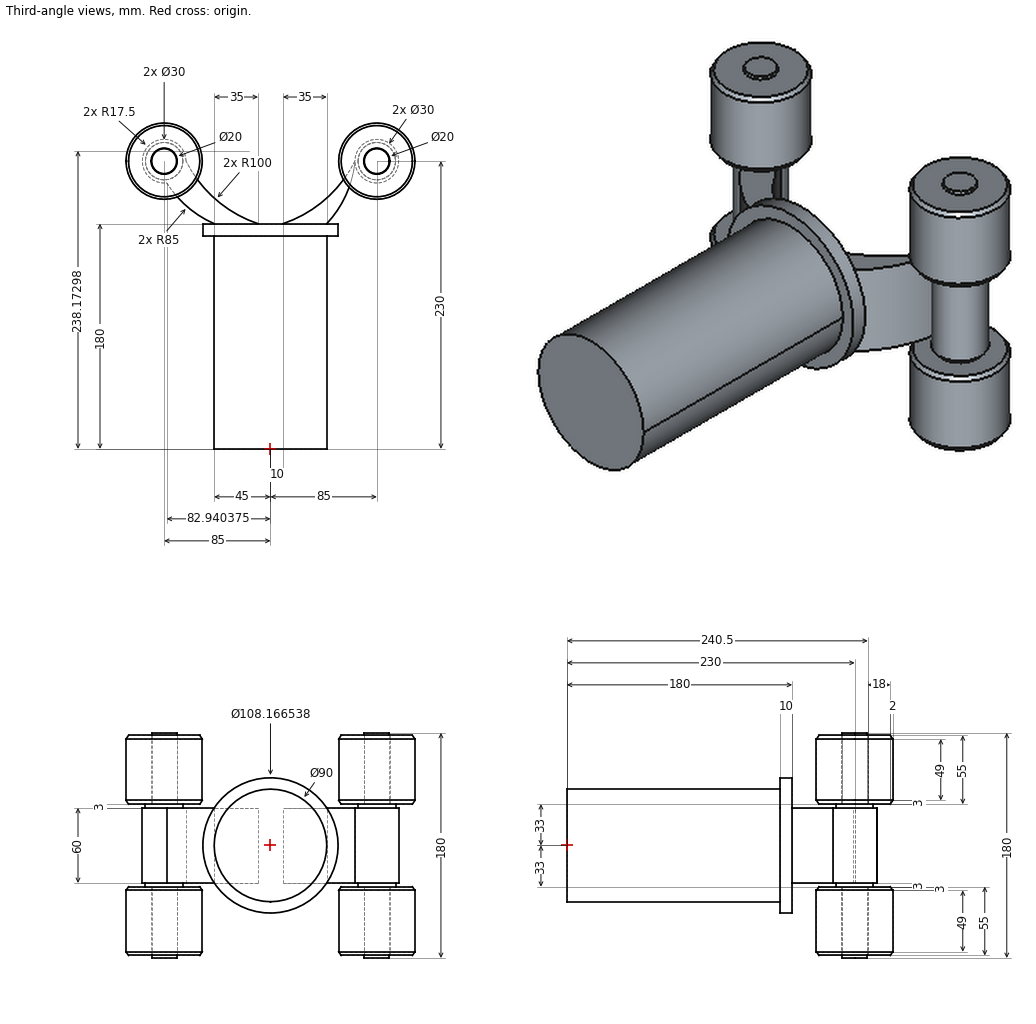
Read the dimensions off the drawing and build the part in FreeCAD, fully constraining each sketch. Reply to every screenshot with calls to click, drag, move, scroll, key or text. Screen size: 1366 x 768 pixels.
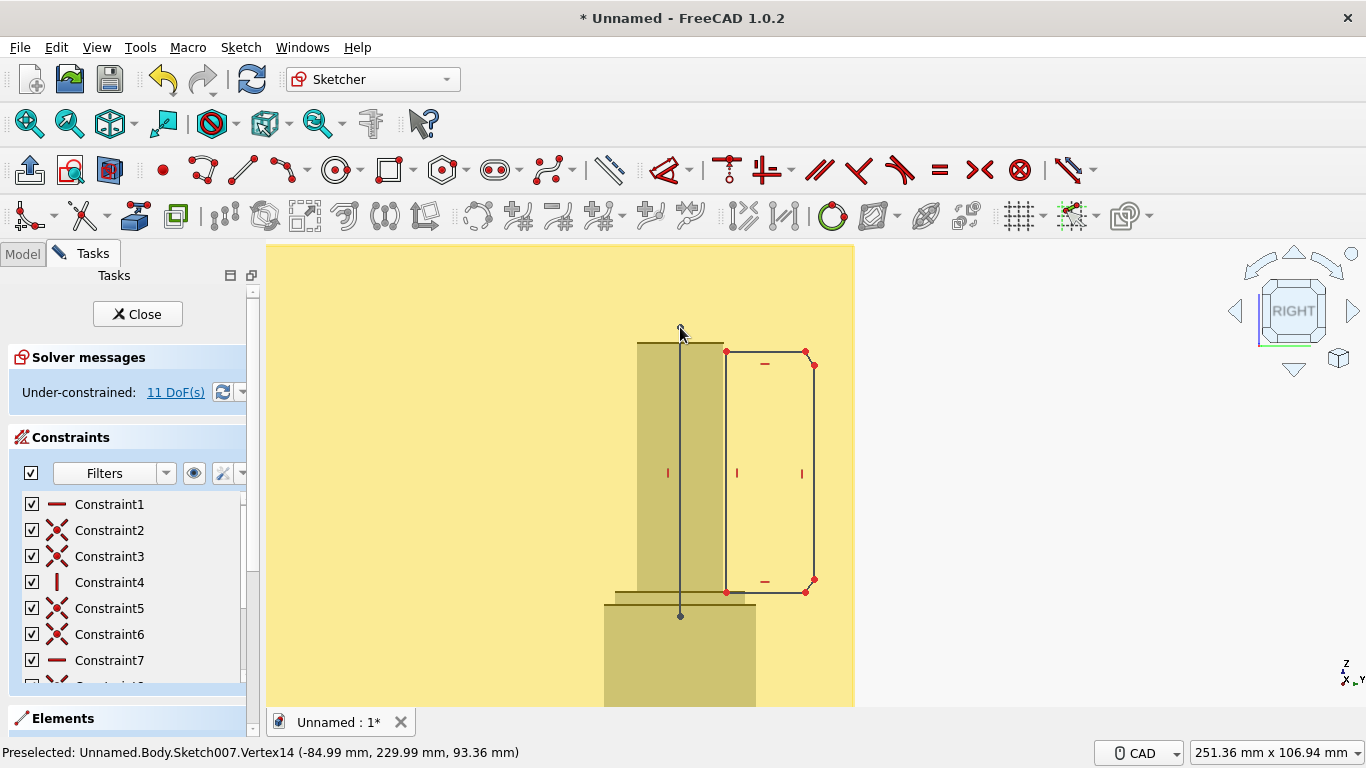
click(680, 530)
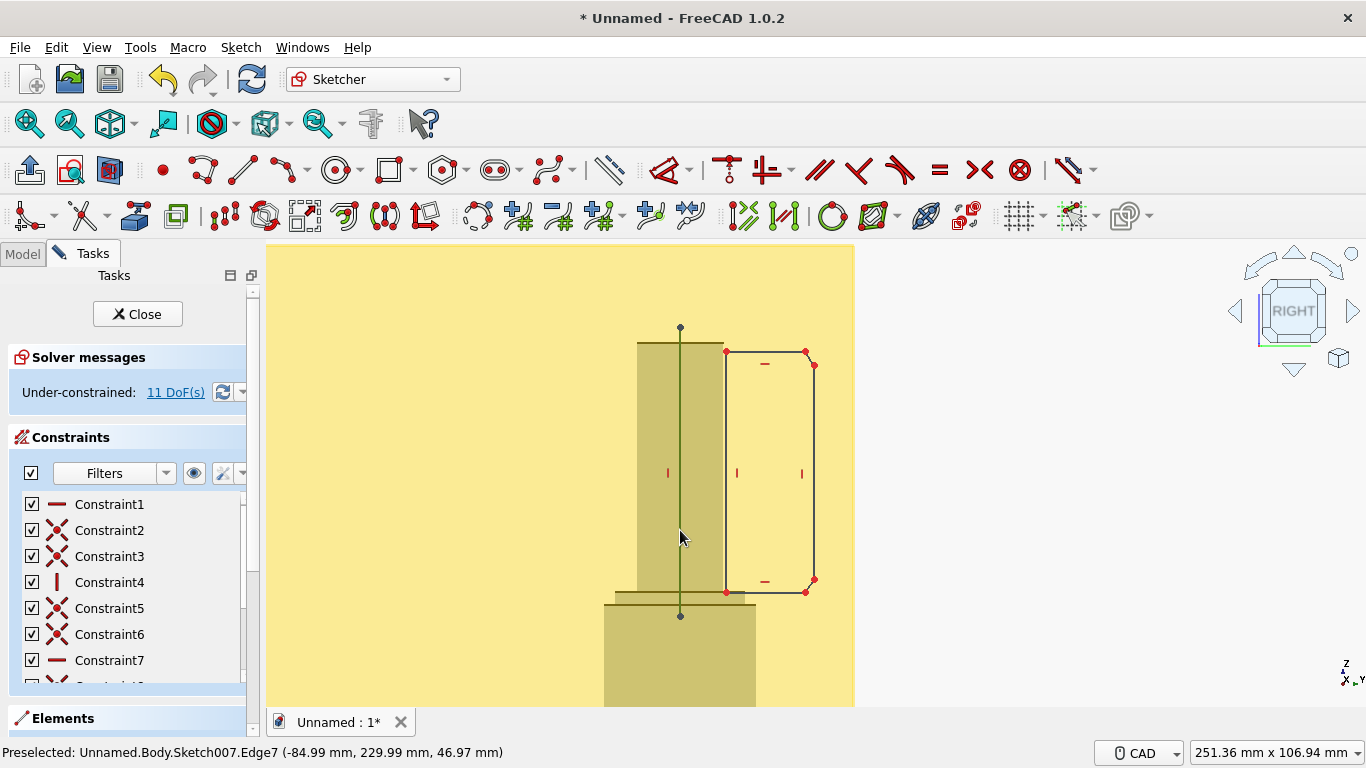
click(610, 170)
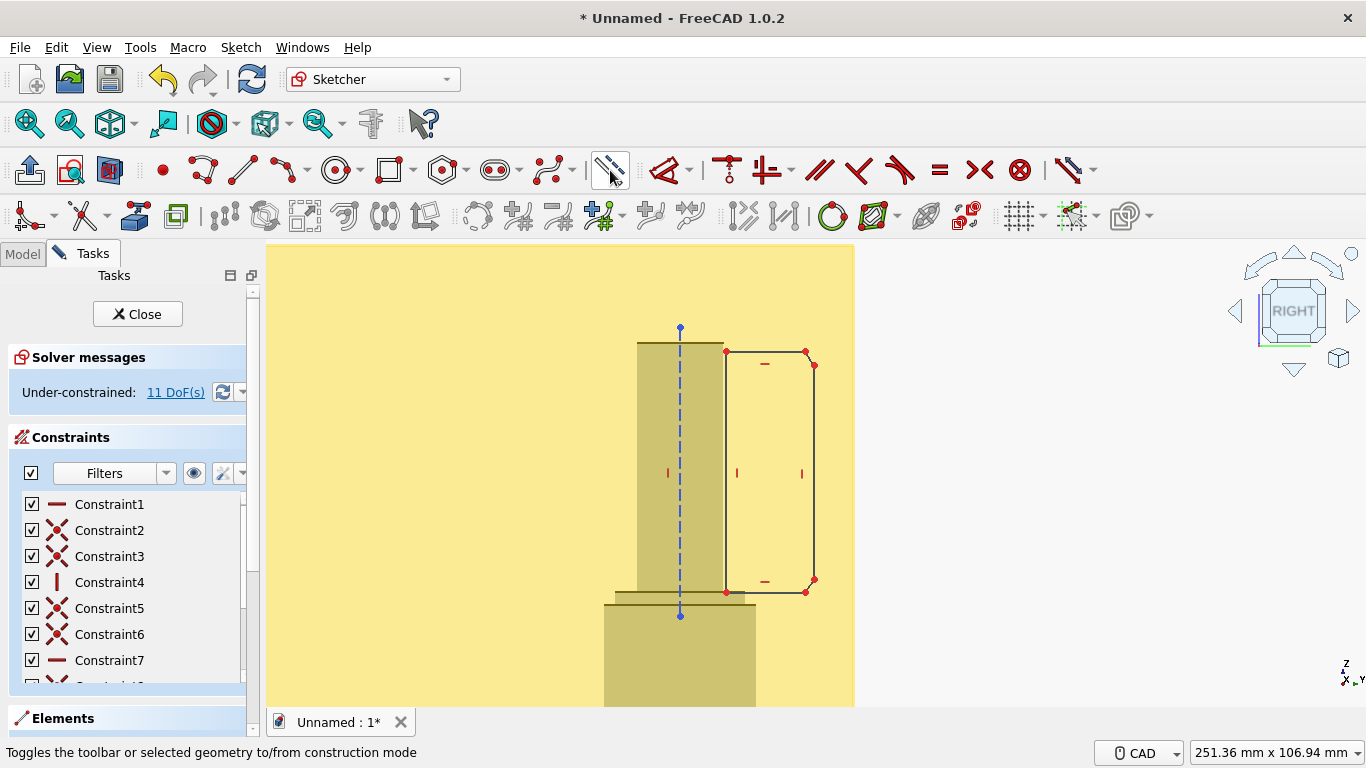
click(664, 170)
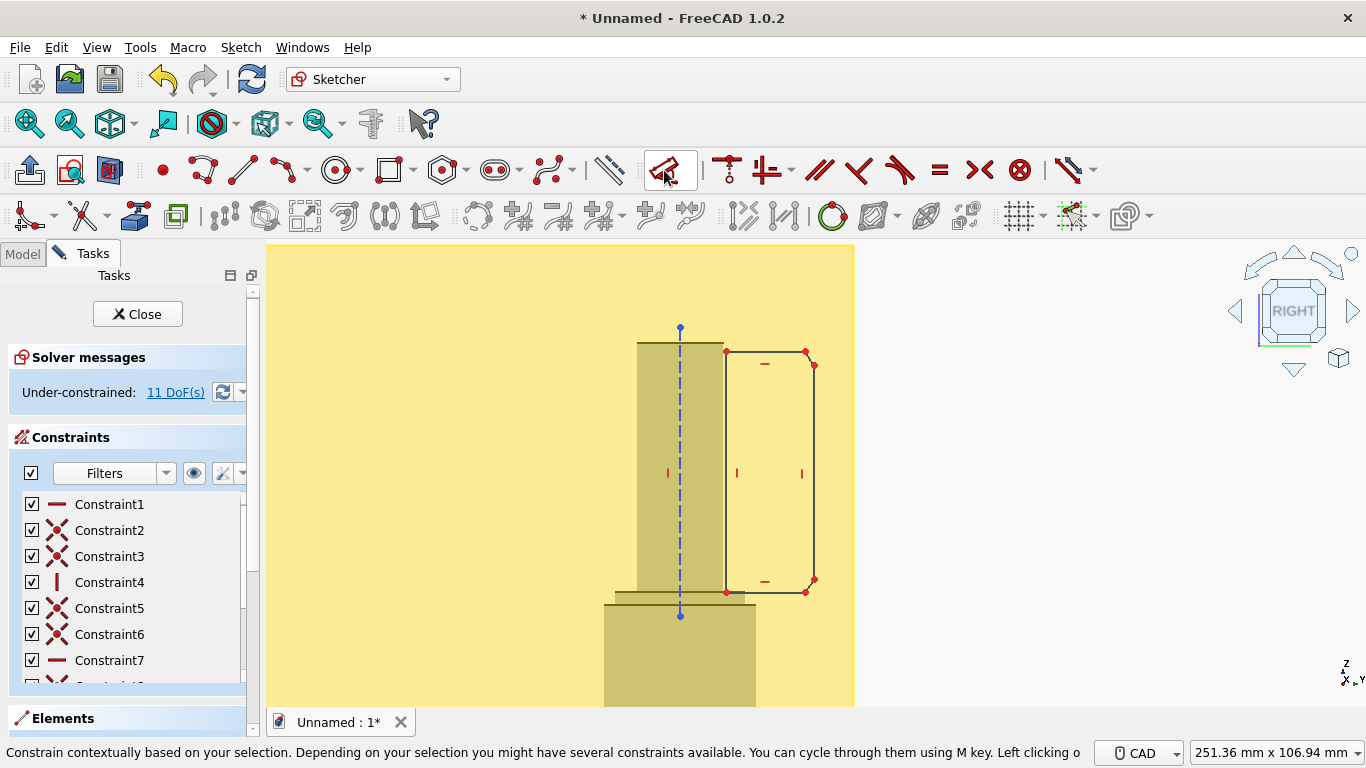
click(750, 593)
click(765, 627)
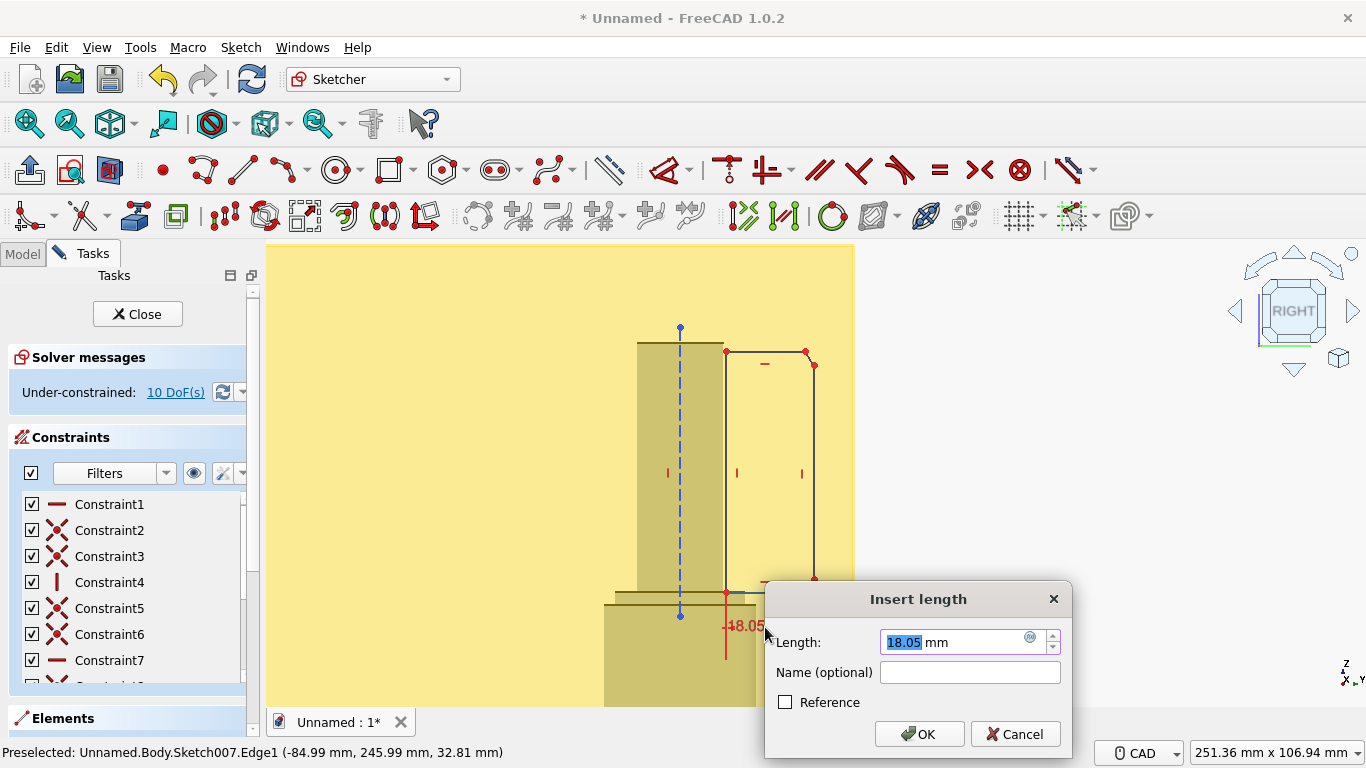
text(18)
key(Return)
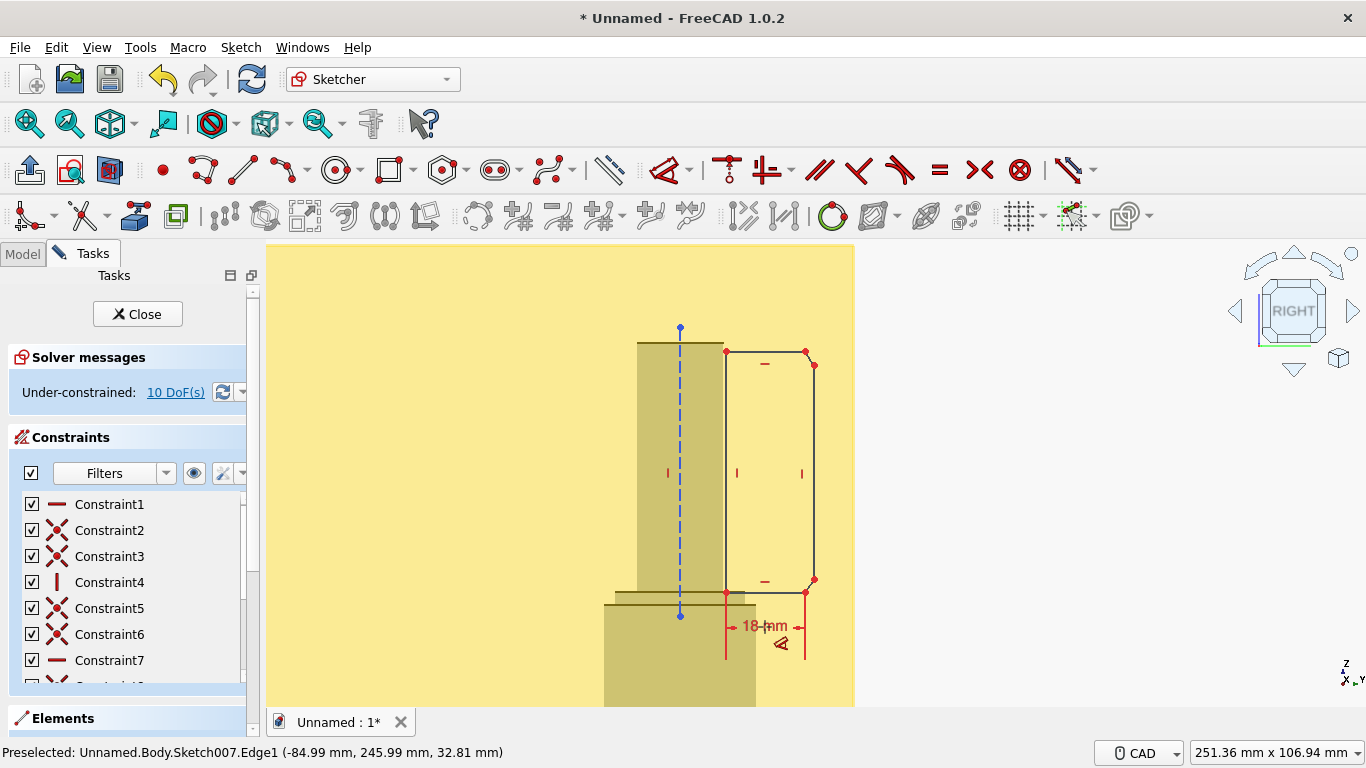
click(814, 516)
click(848, 473)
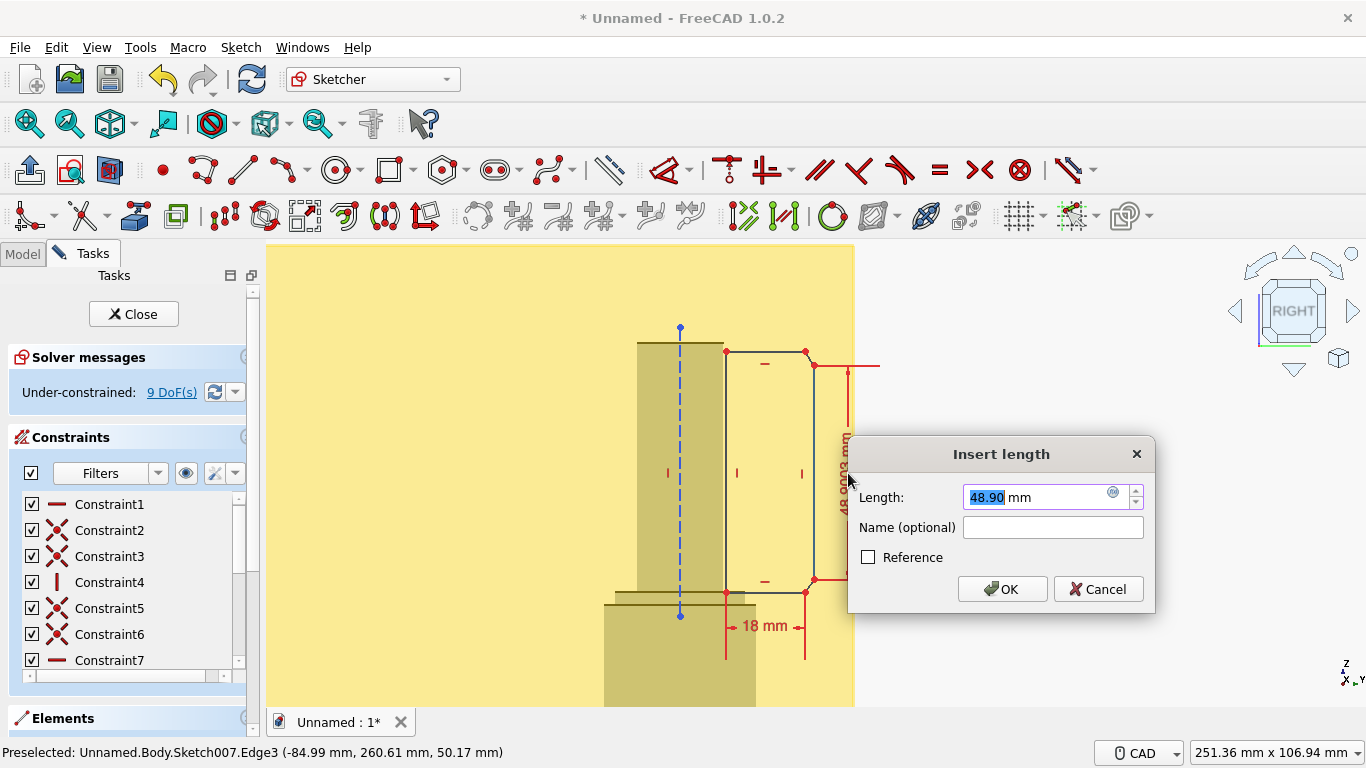
text(49)
key(Return)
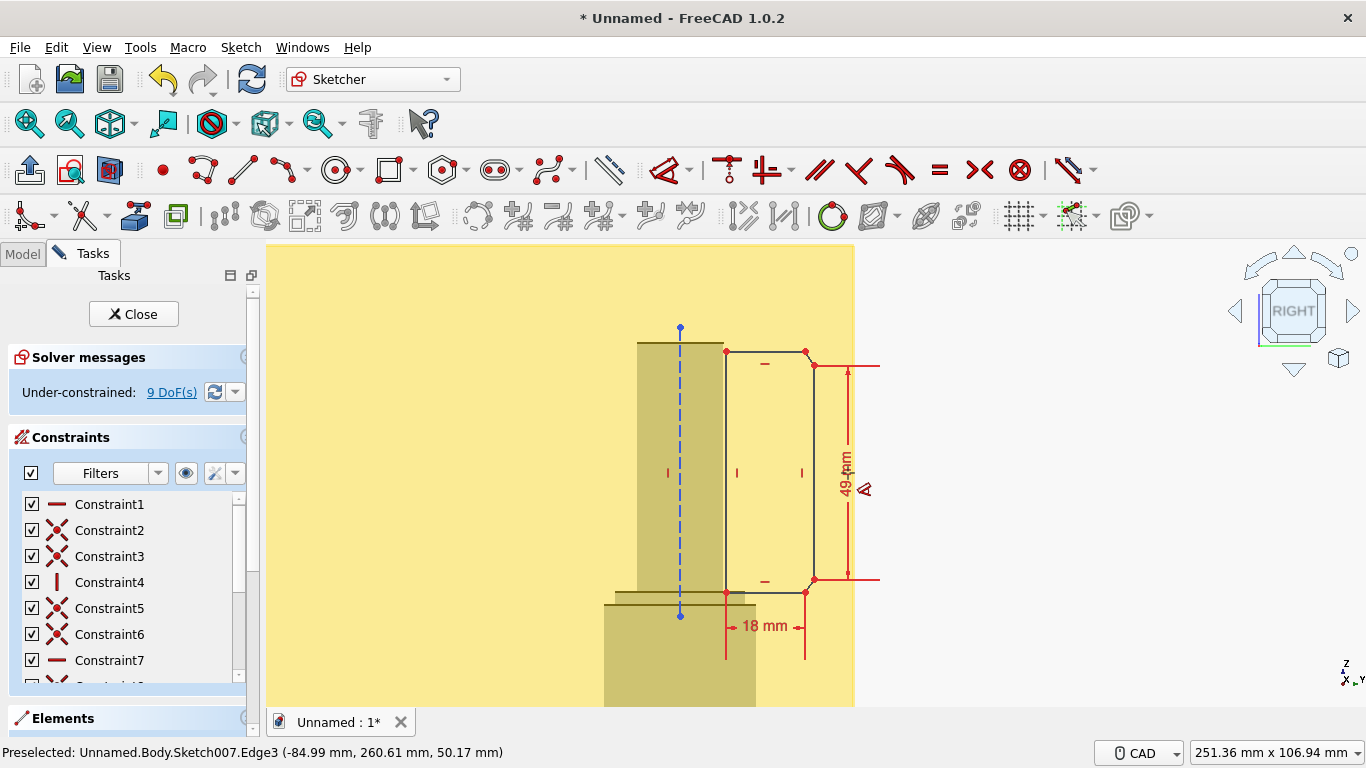
click(781, 352)
click(766, 318)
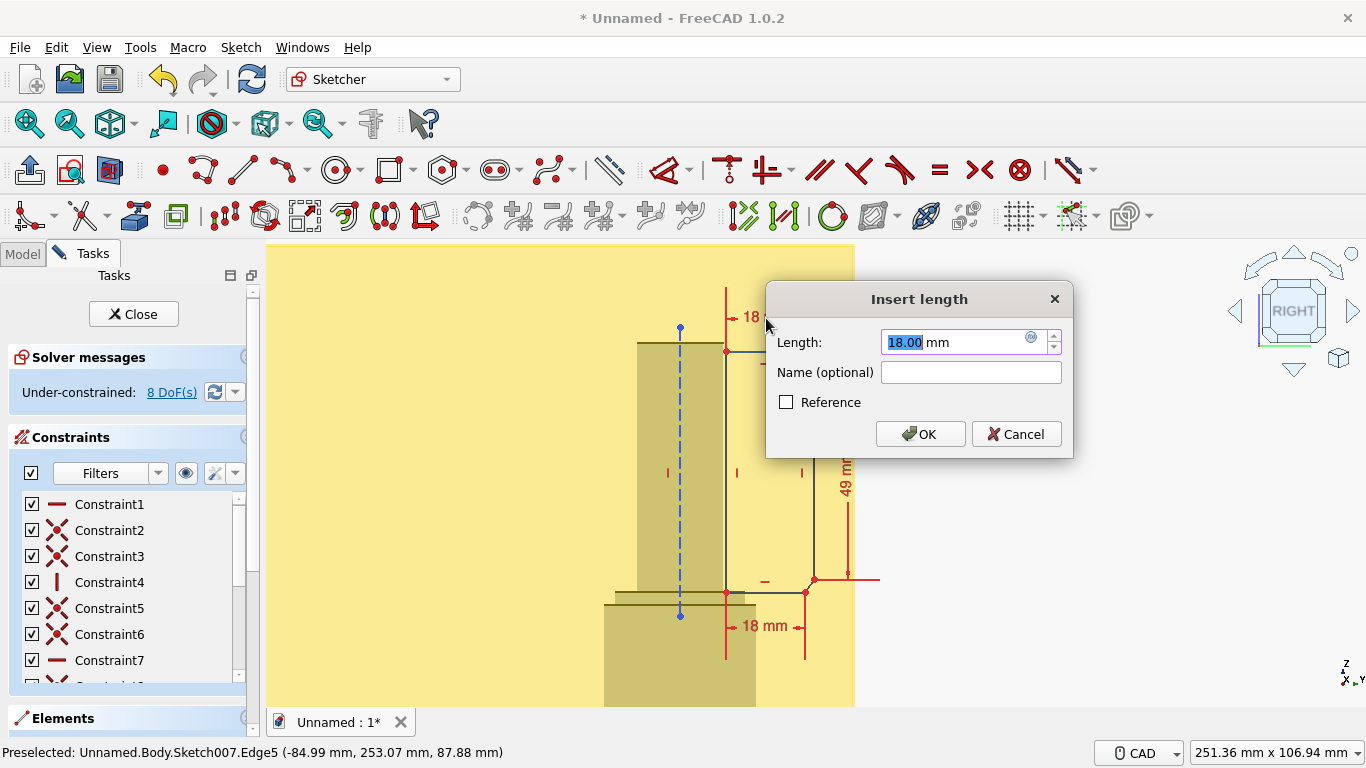
text(18)
key(Return)